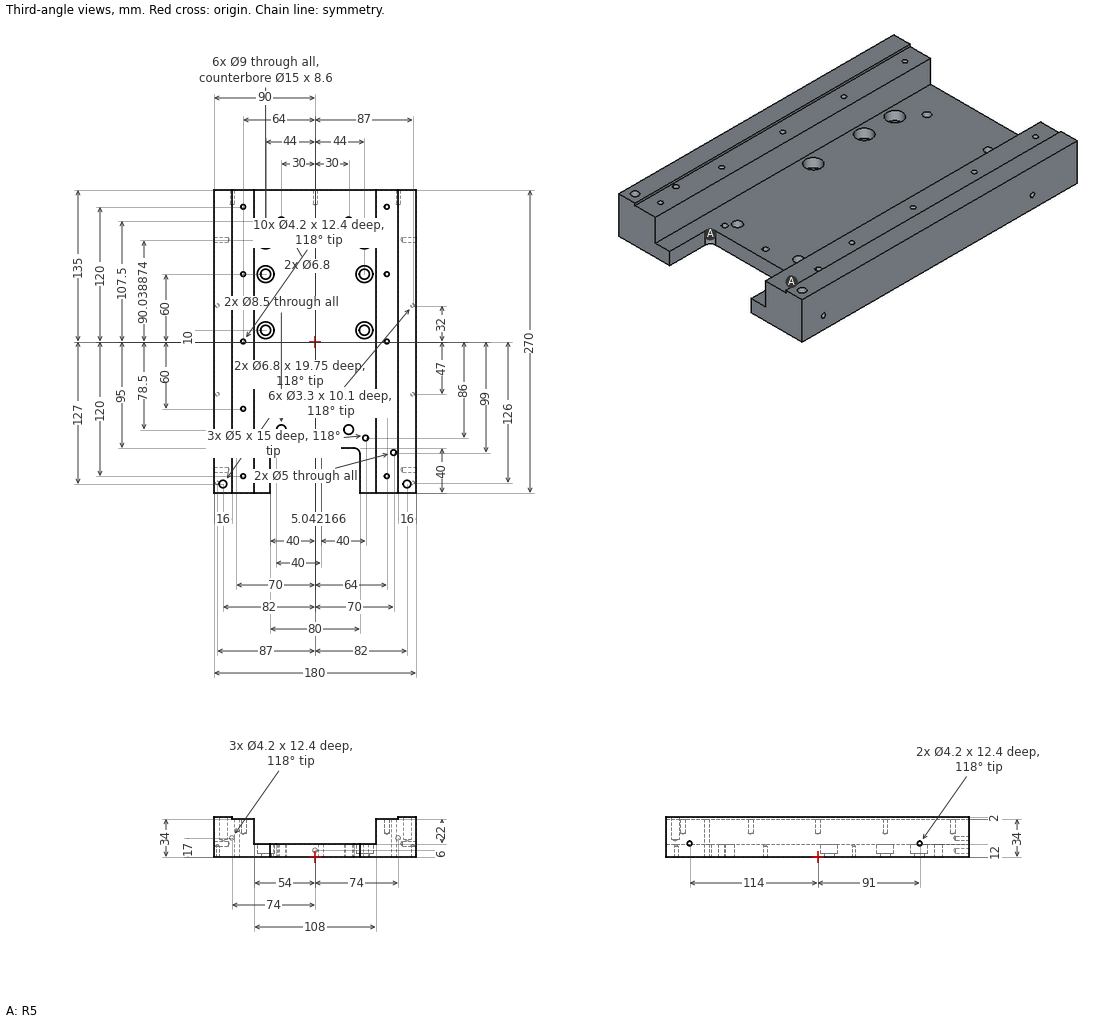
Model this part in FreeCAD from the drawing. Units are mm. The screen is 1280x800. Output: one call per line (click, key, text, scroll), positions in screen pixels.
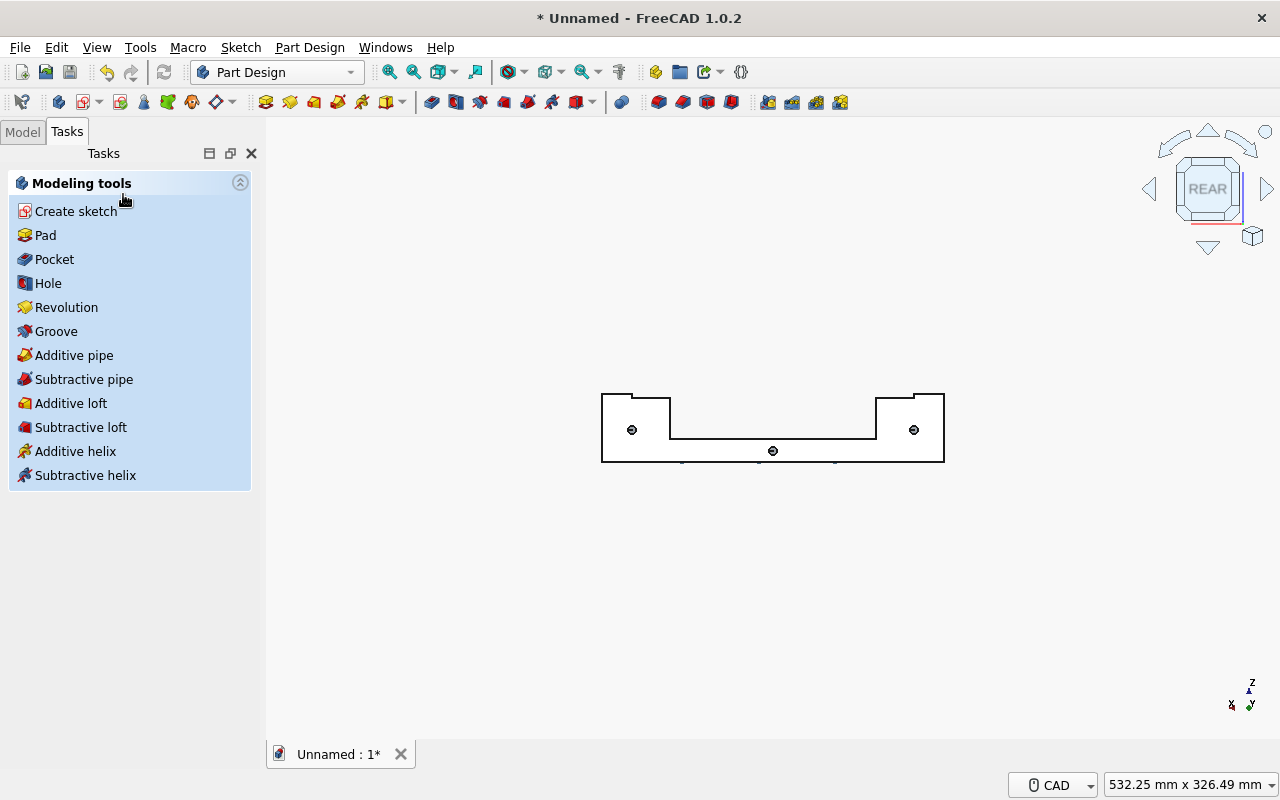
click(456, 102)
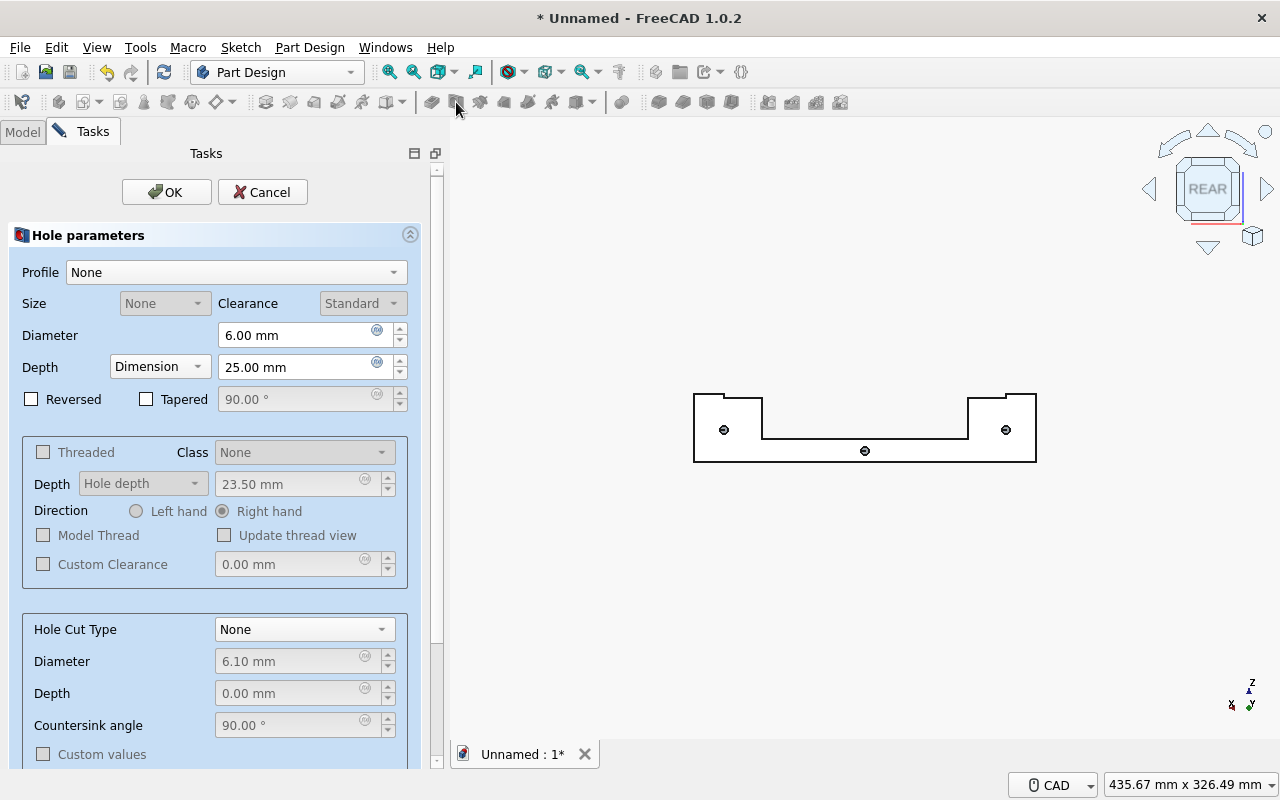
triple_click(305, 335)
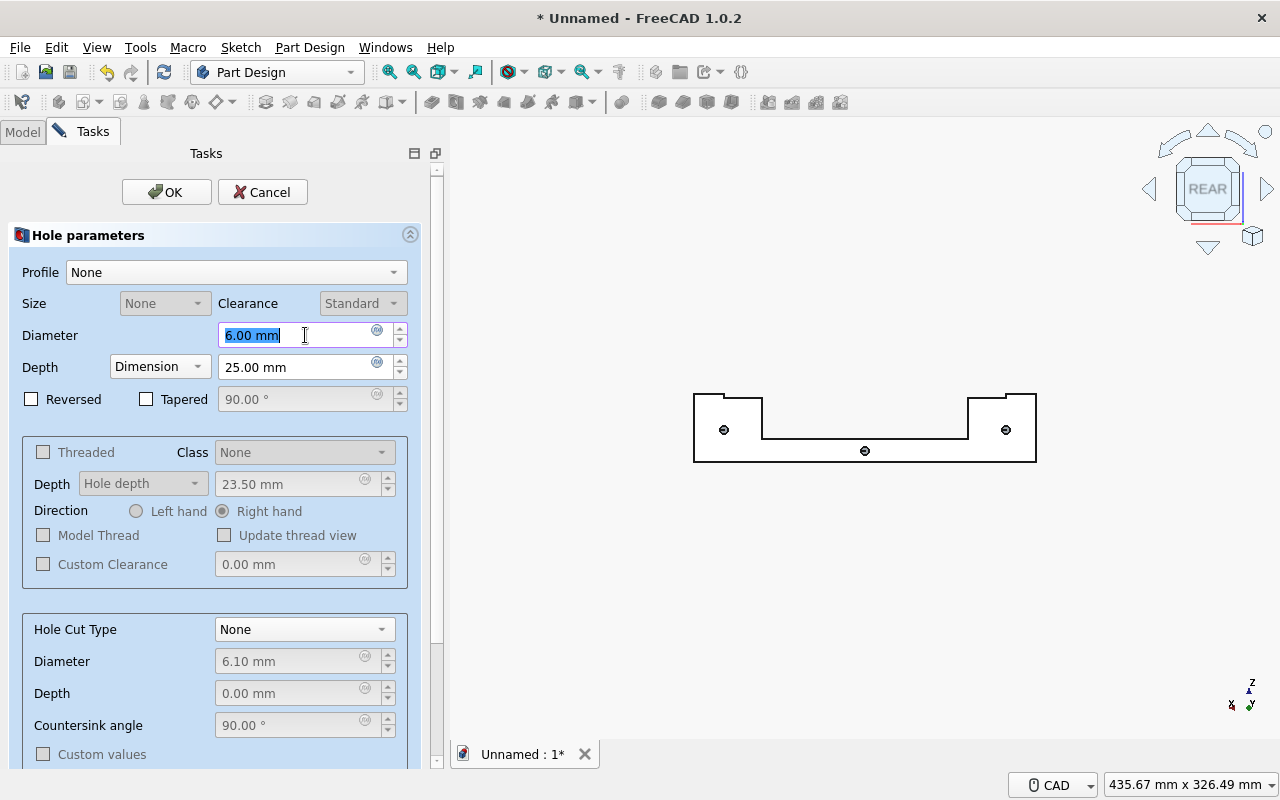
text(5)
key(Tab)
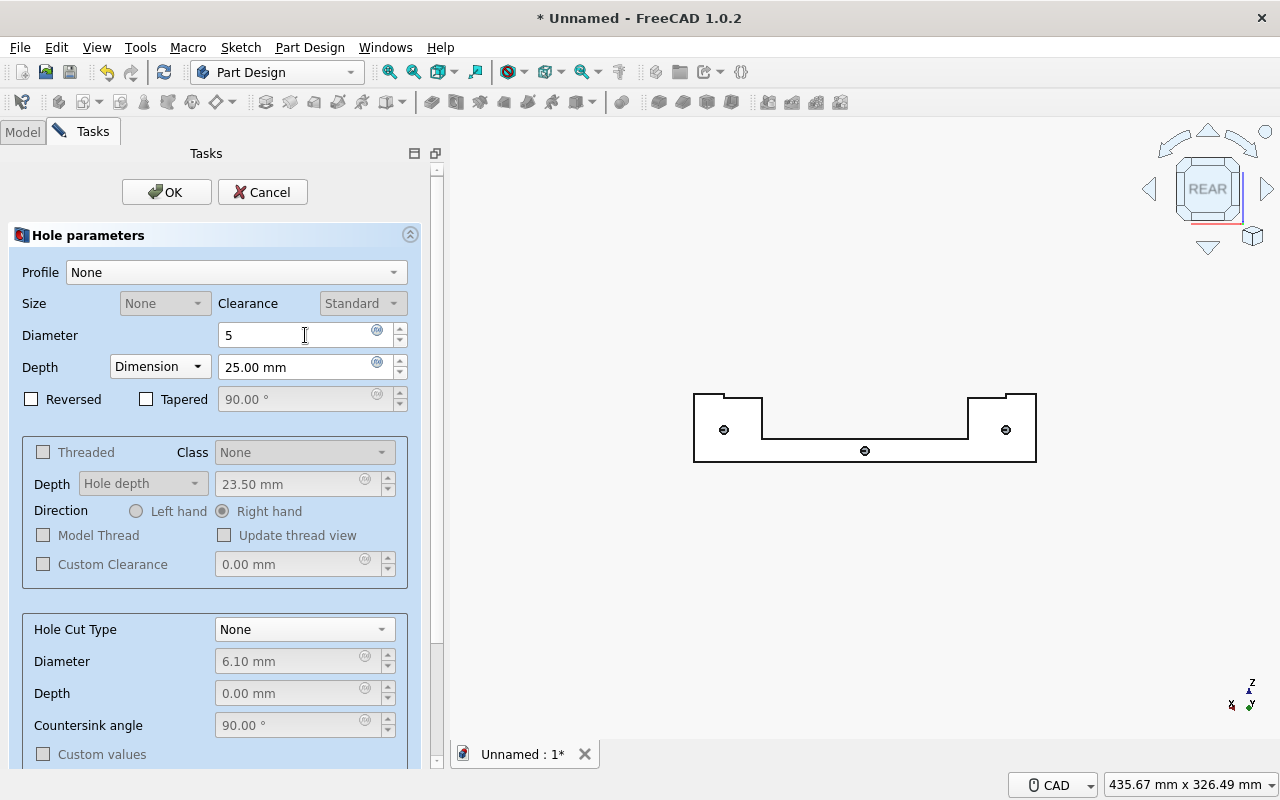
triple_click(305, 367)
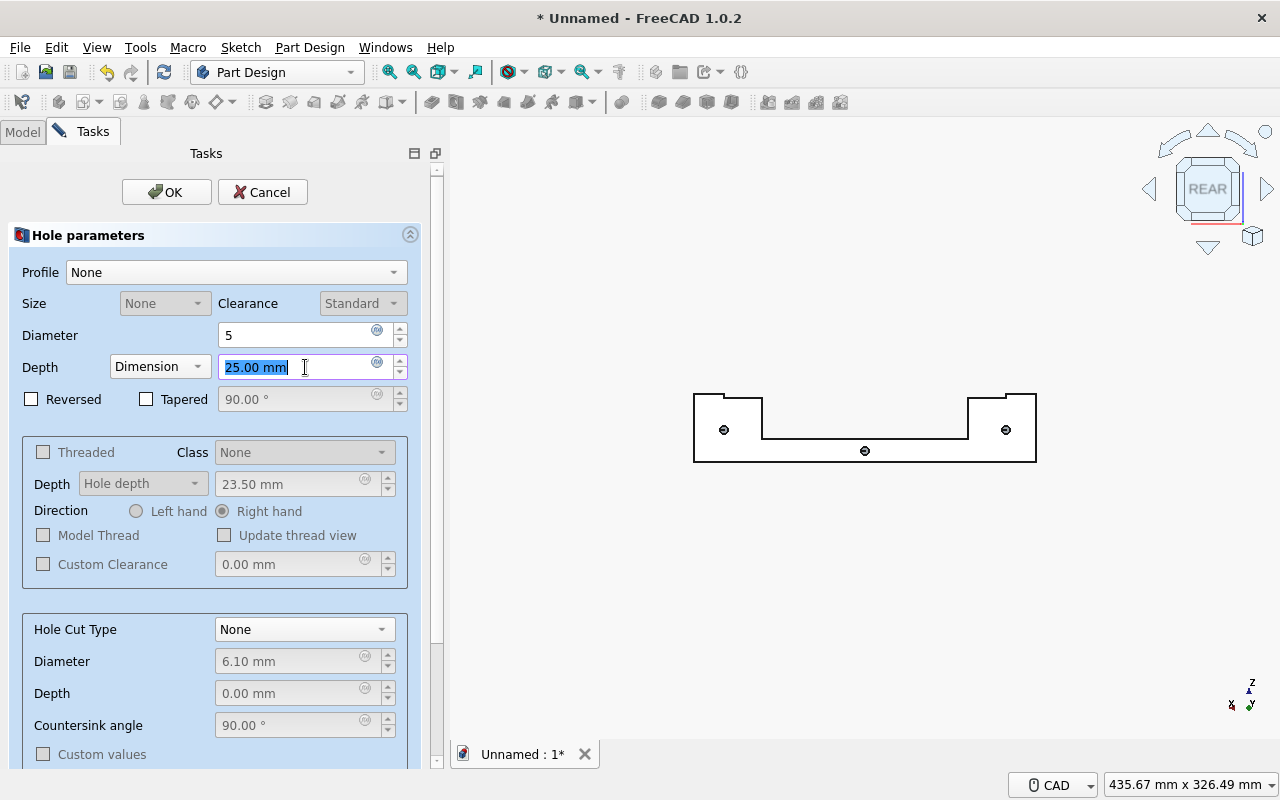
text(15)
key(Tab)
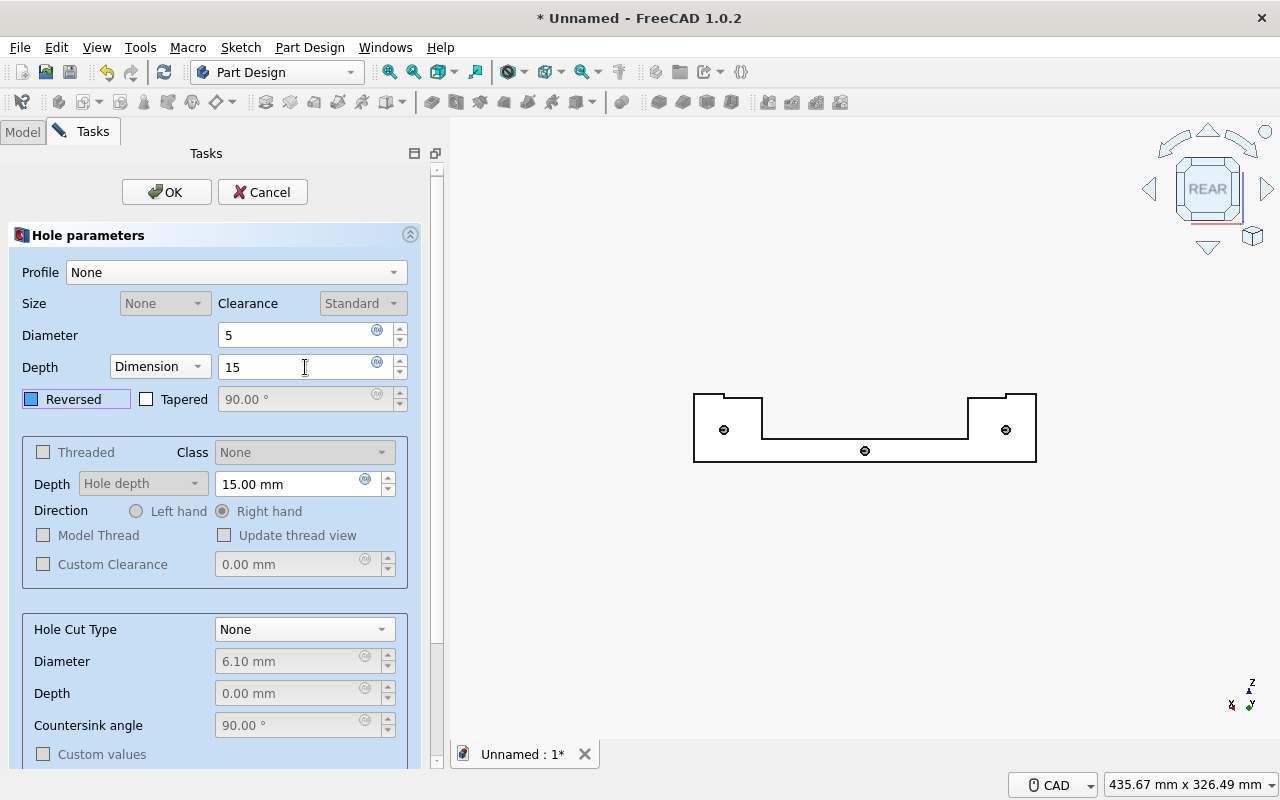
click(30, 399)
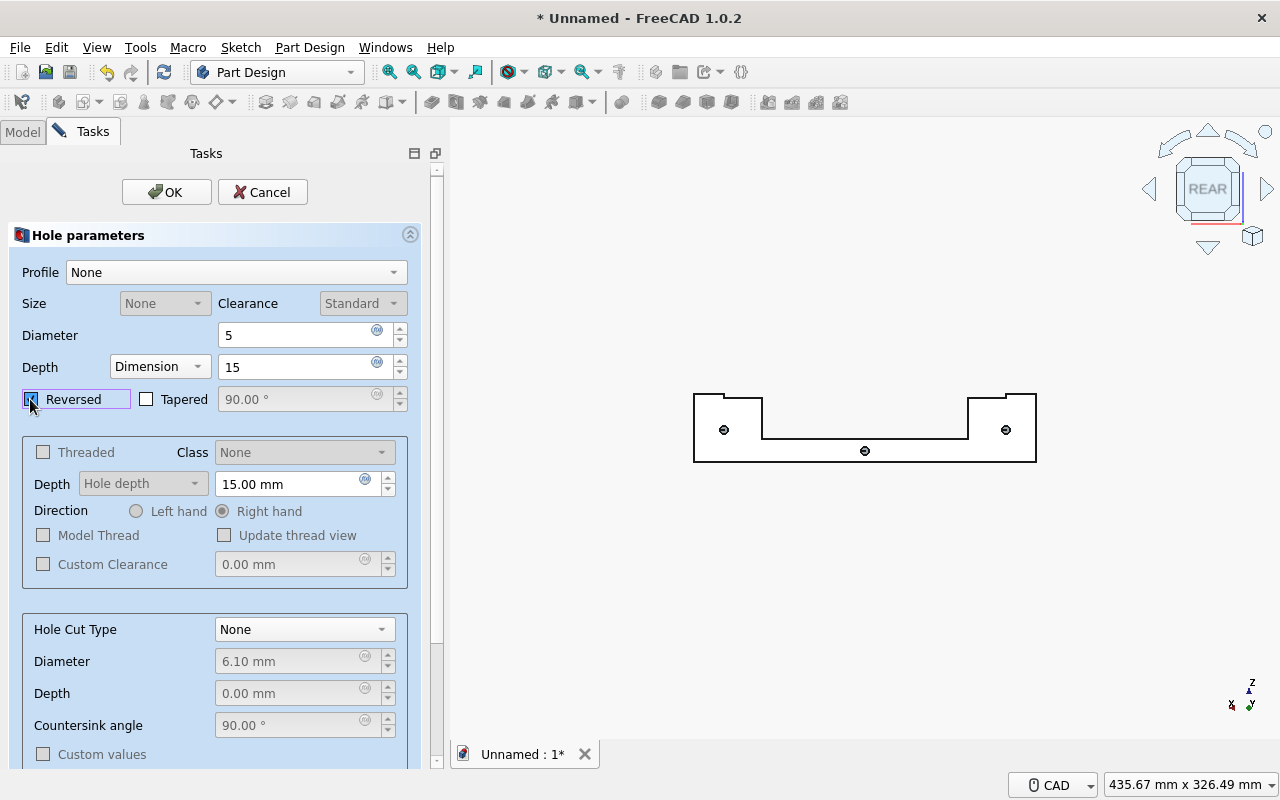
click(167, 192)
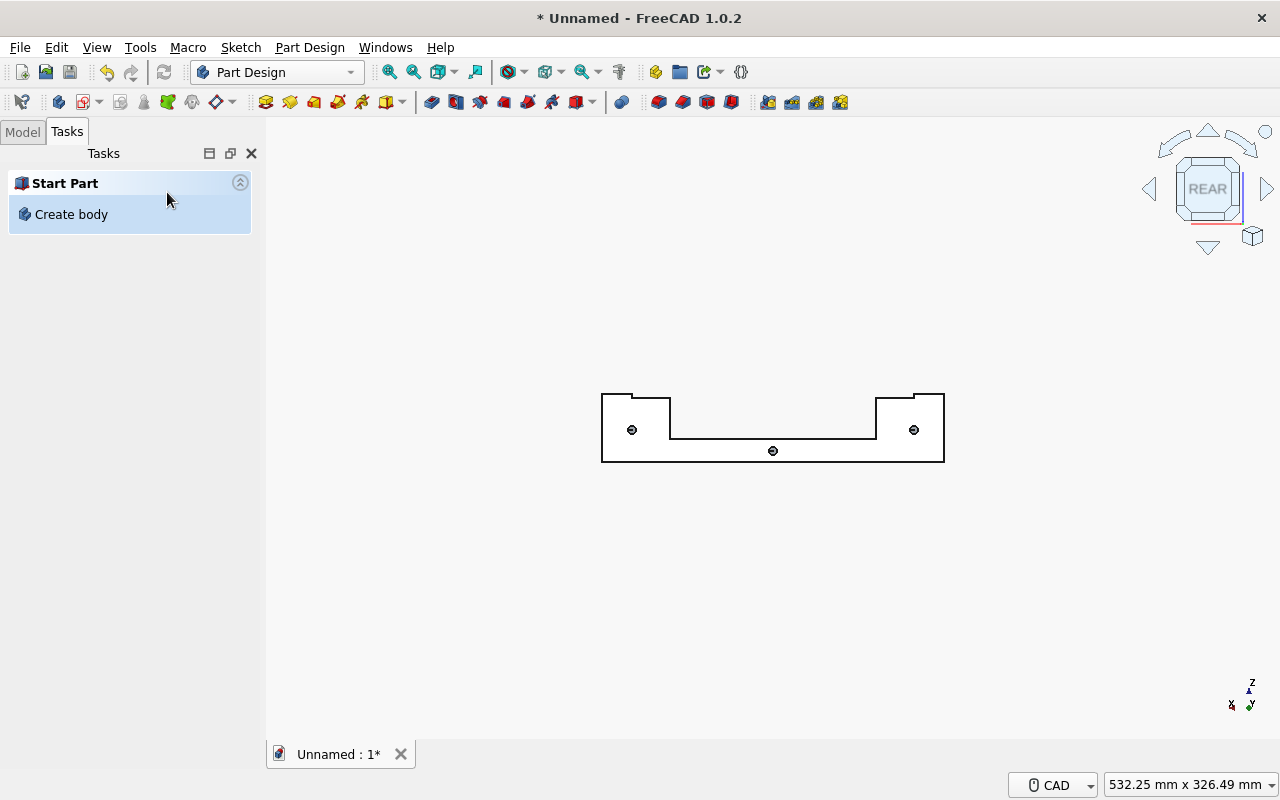
key(v)
key(f)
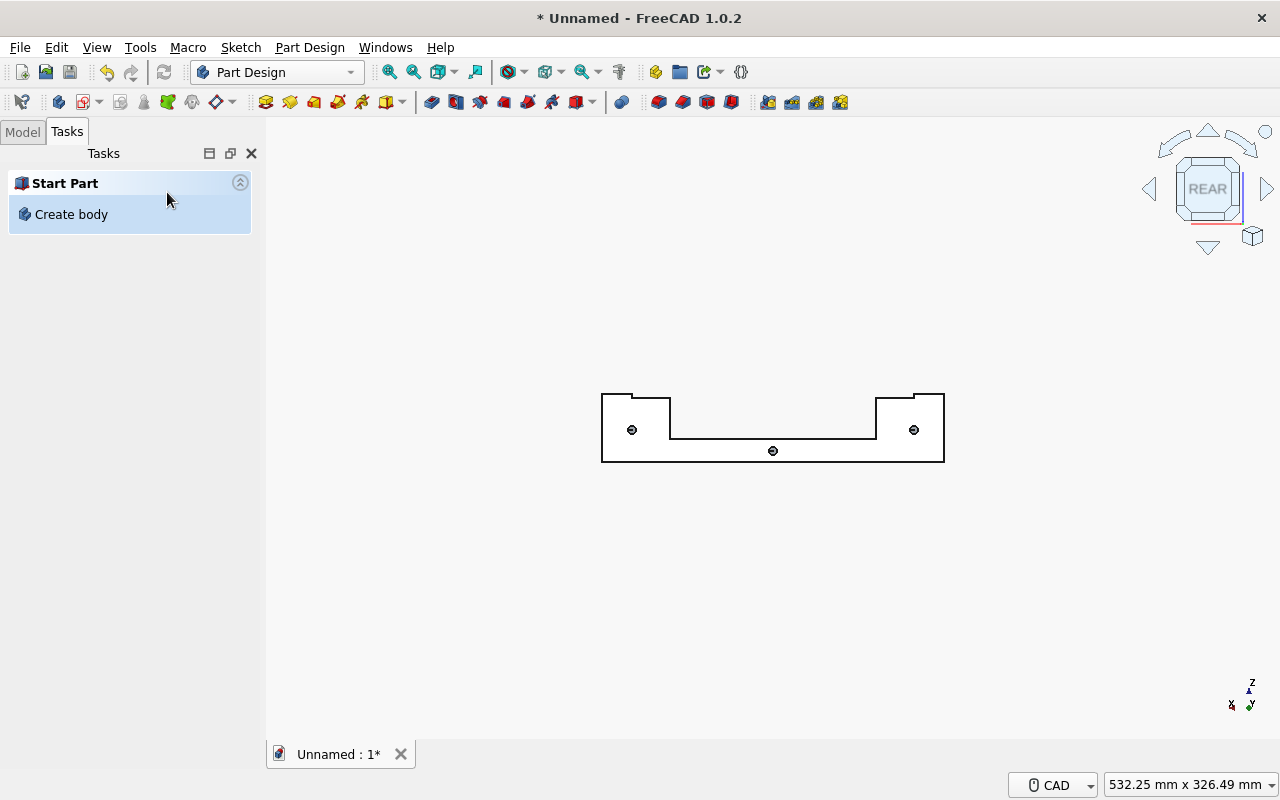
key(0)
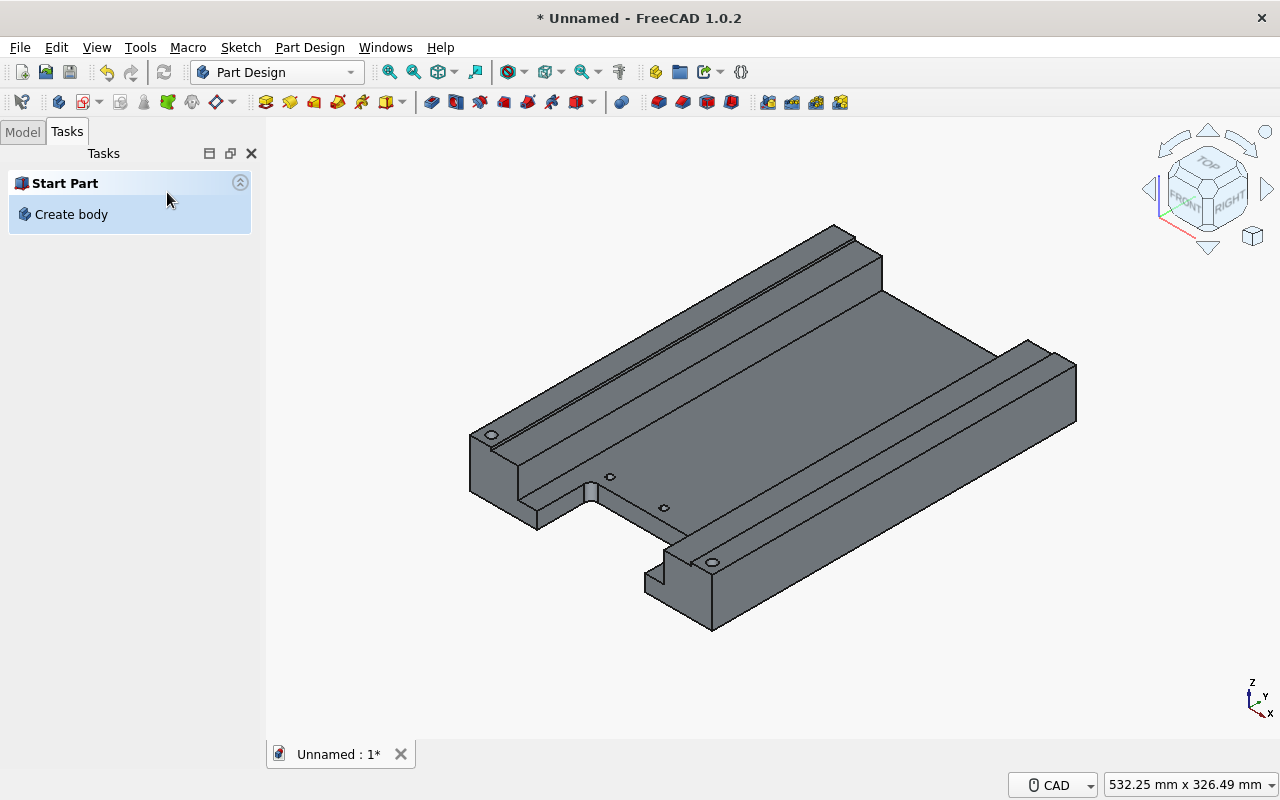
click(877, 376)